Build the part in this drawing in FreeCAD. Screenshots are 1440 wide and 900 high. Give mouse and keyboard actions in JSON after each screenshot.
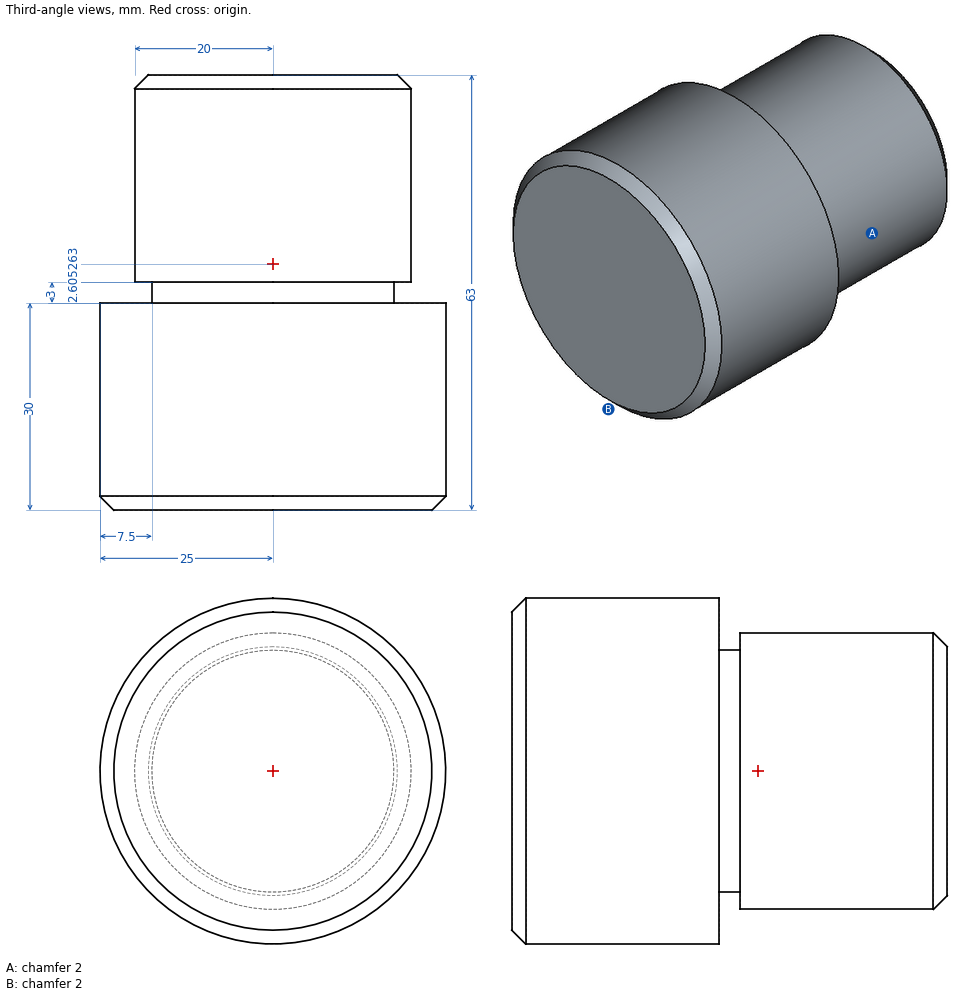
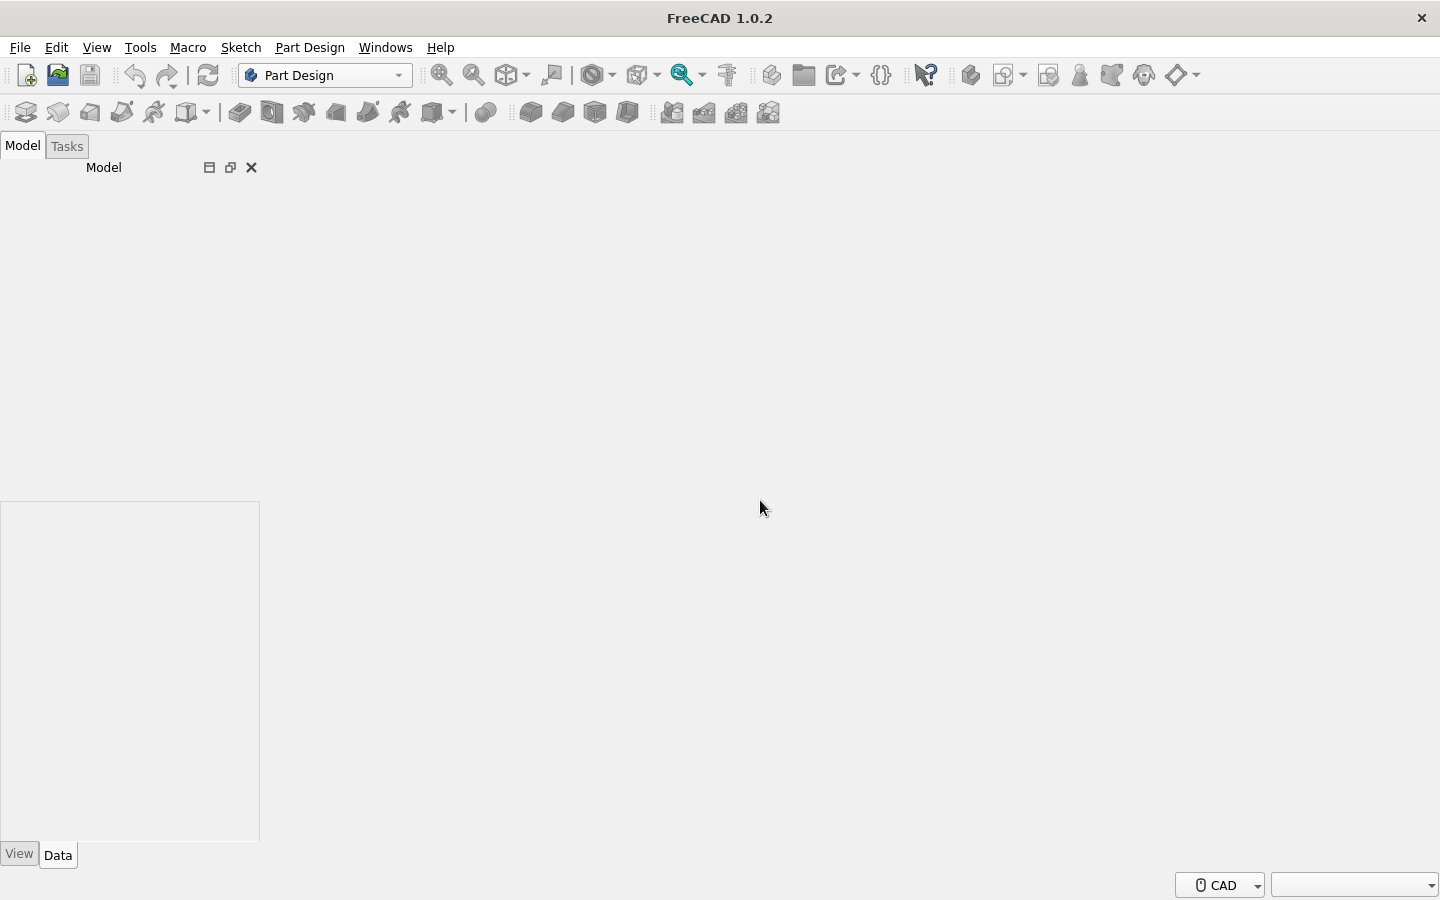
{"action": "left_click", "coordinate": [26, 76]}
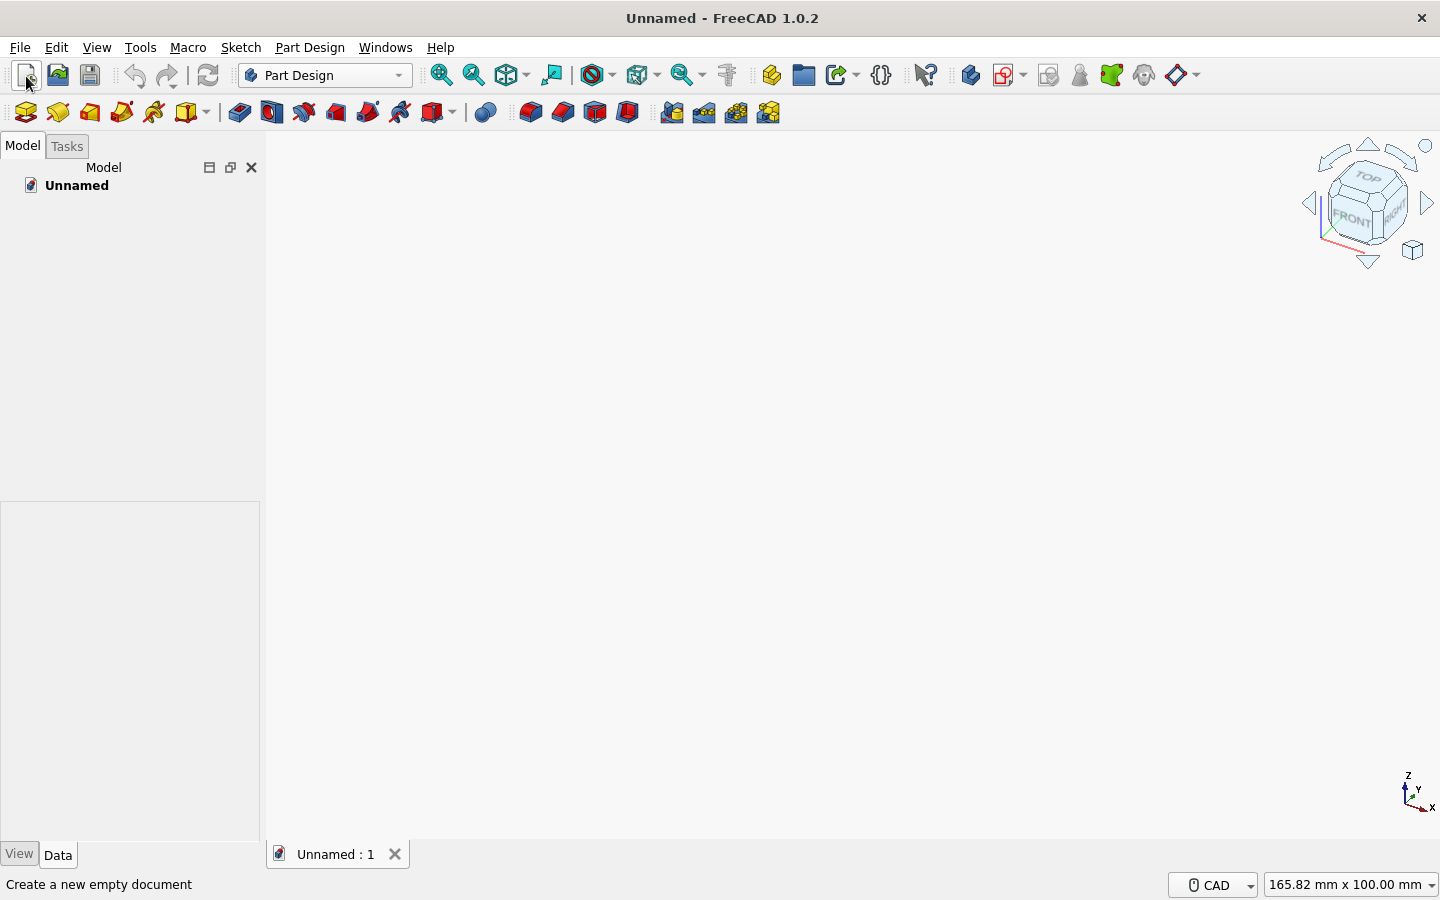
{"action": "left_click", "coordinate": [1004, 76]}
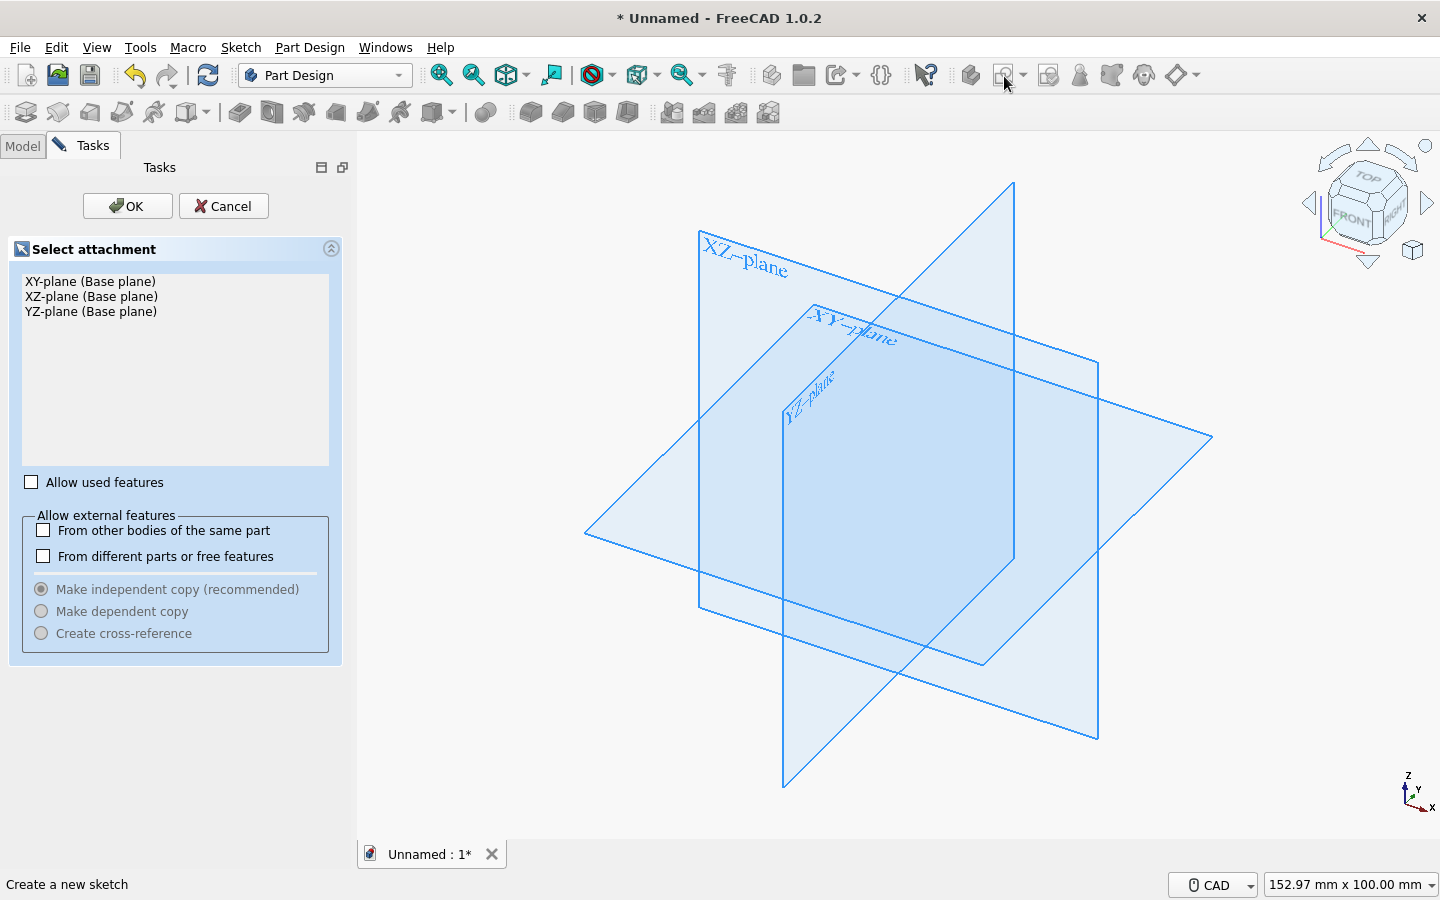
{"action": "left_click", "coordinate": [82, 282]}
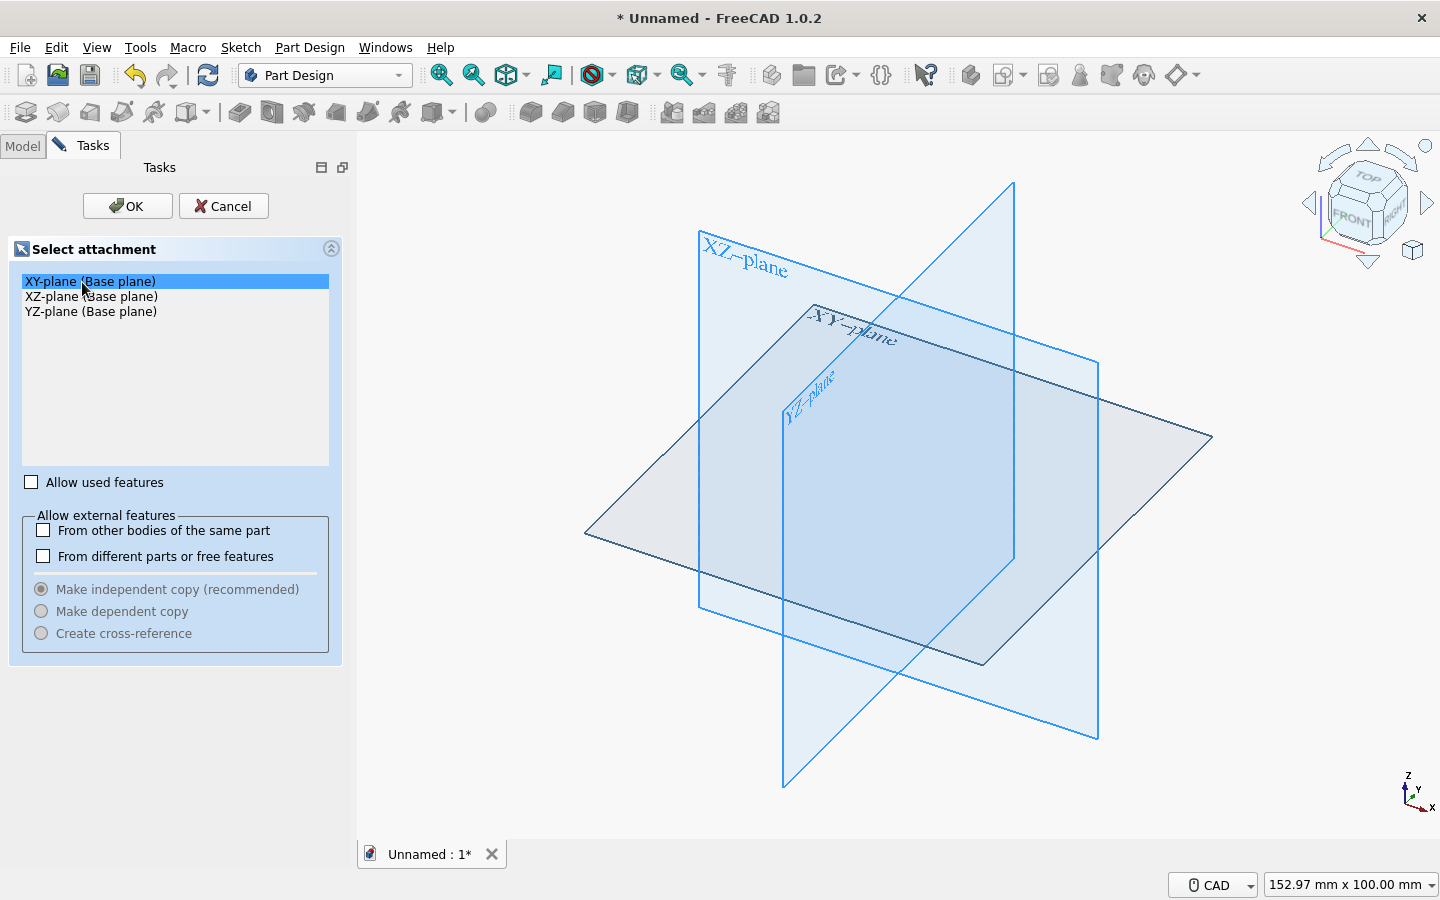
{"action": "left_click", "coordinate": [128, 206]}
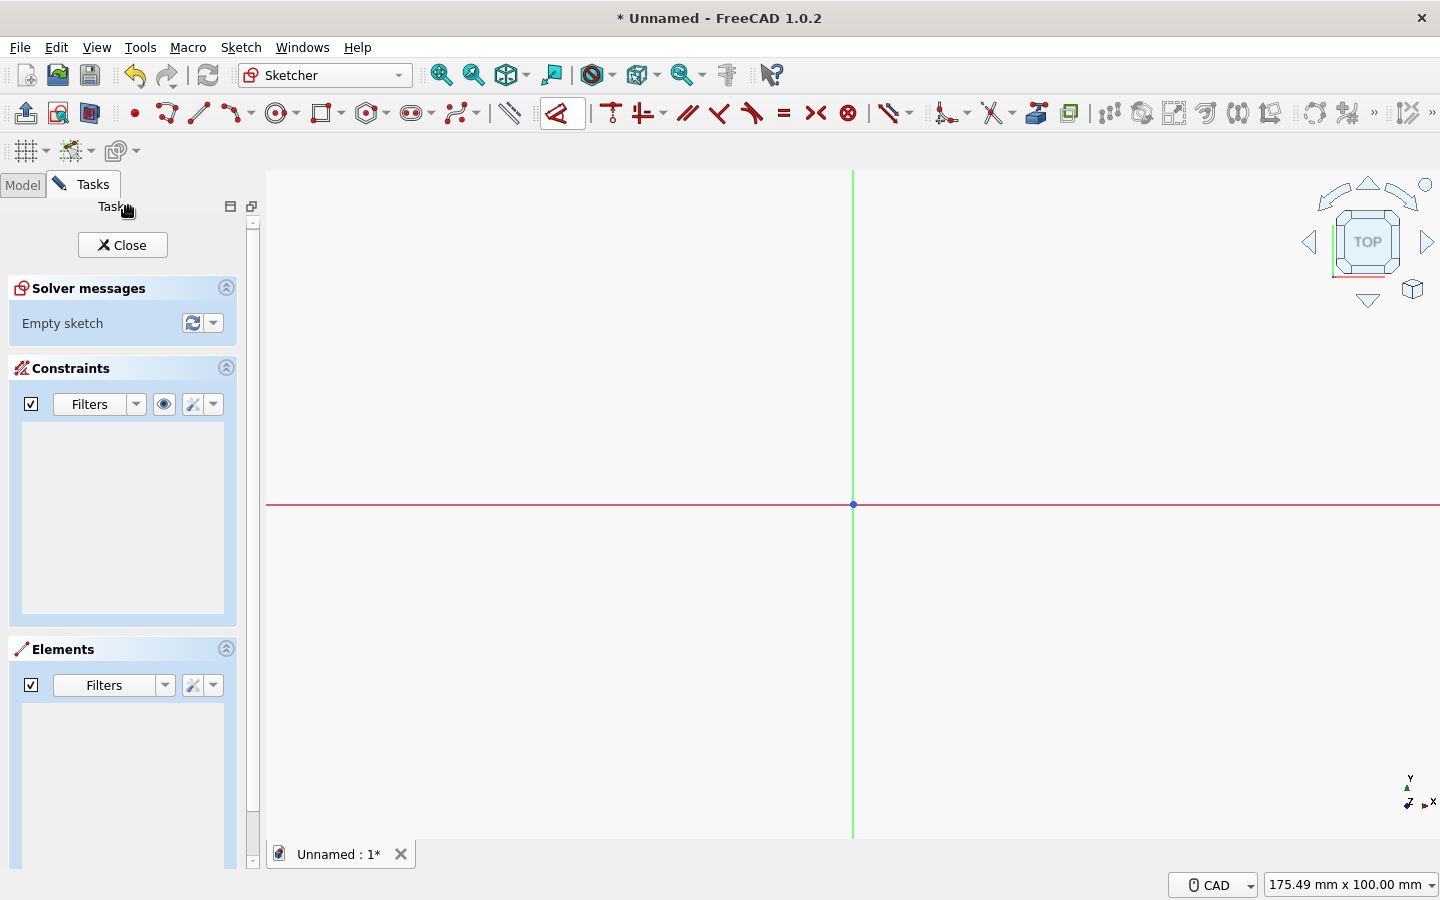
{"action": "key", "text": "g m"}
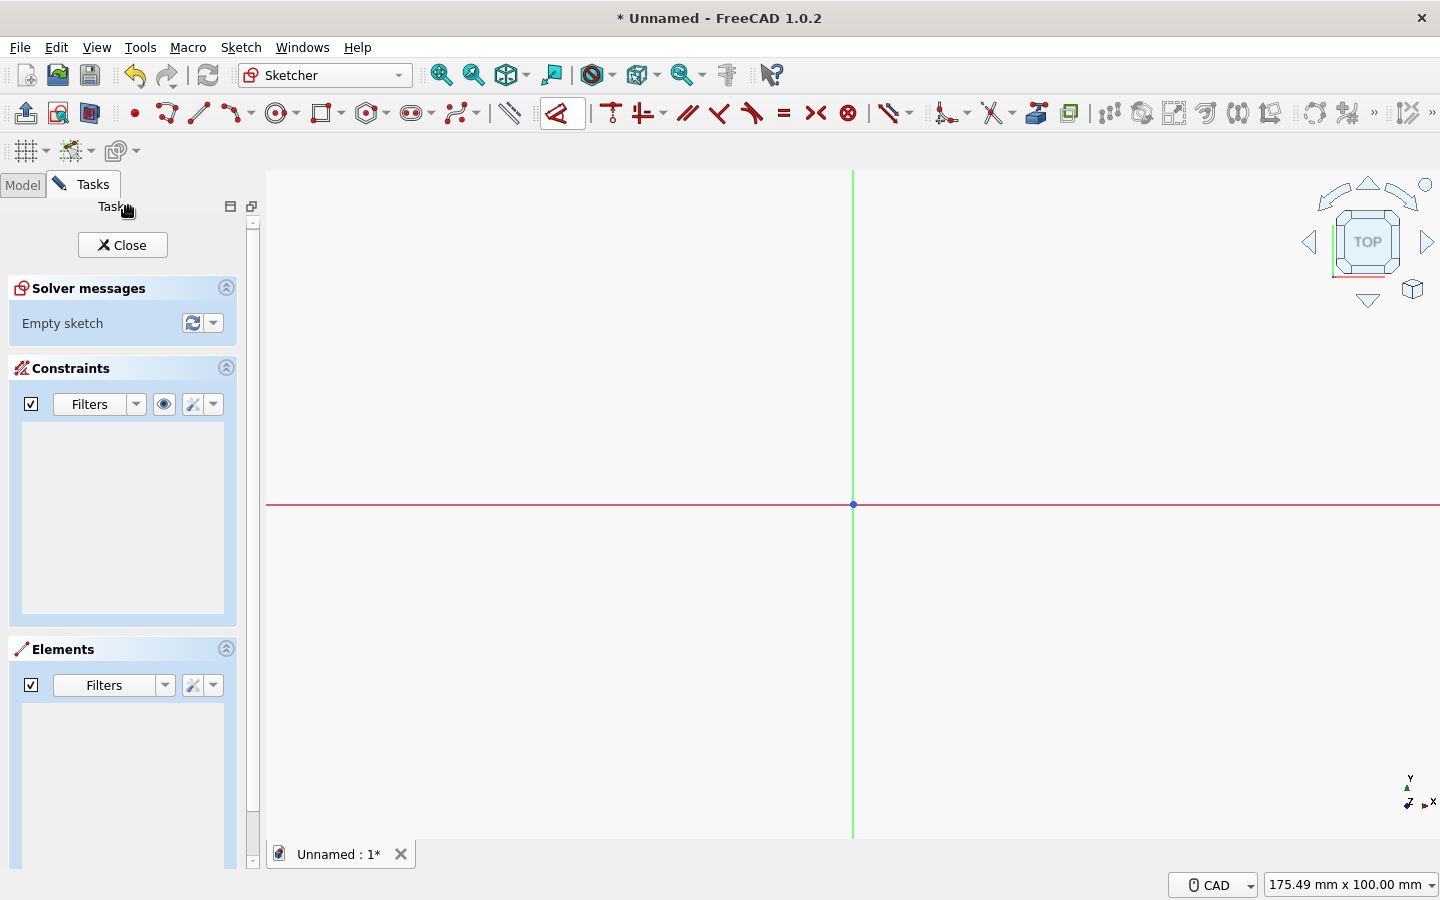
{"action": "left_click", "coordinate": [736, 522]}
{"action": "left_click", "coordinate": [736, 542]}
{"action": "left_click", "coordinate": [686, 542]}
{"action": "left_click", "coordinate": [686, 743]}
{"action": "left_click", "coordinate": [853, 743]}
{"action": "left_click", "coordinate": [844, 321]}
{"action": "left_click", "coordinate": [719, 321]}
{"action": "left_click", "coordinate": [719, 522]}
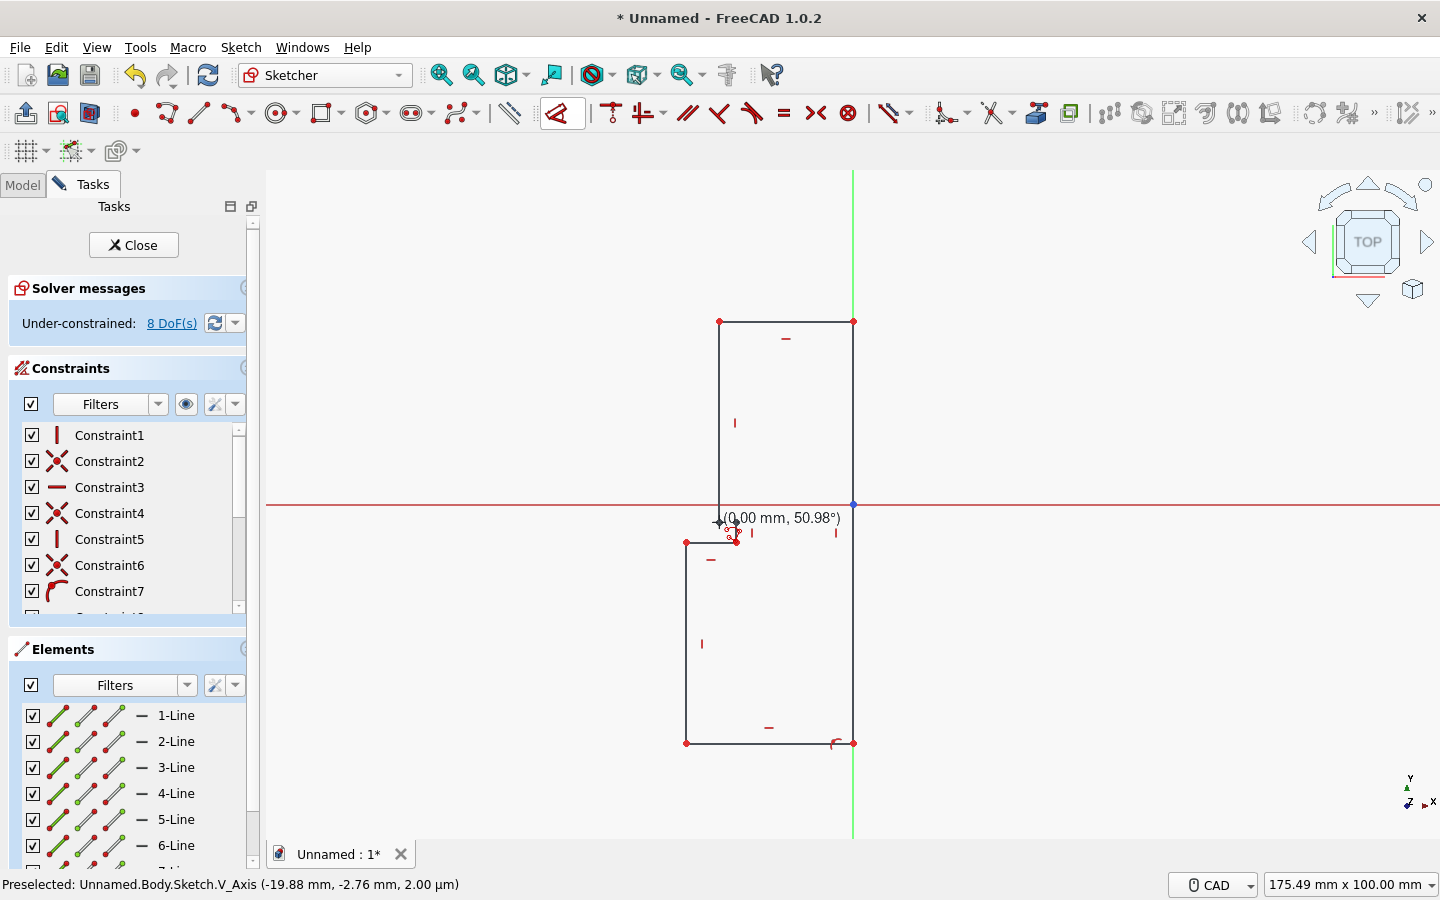
{"action": "scroll", "coordinate": [736, 522], "scroll_direction": "up", "scroll_amount": 3}